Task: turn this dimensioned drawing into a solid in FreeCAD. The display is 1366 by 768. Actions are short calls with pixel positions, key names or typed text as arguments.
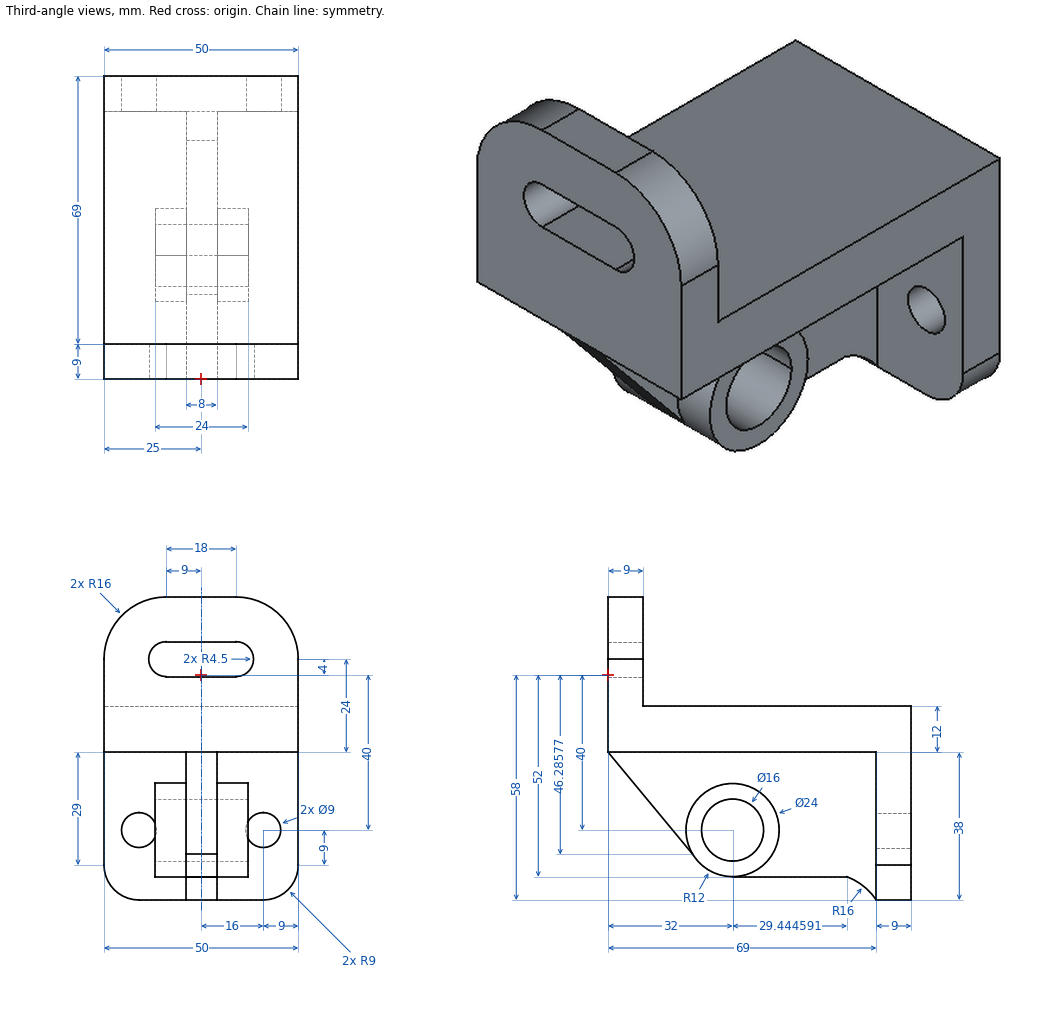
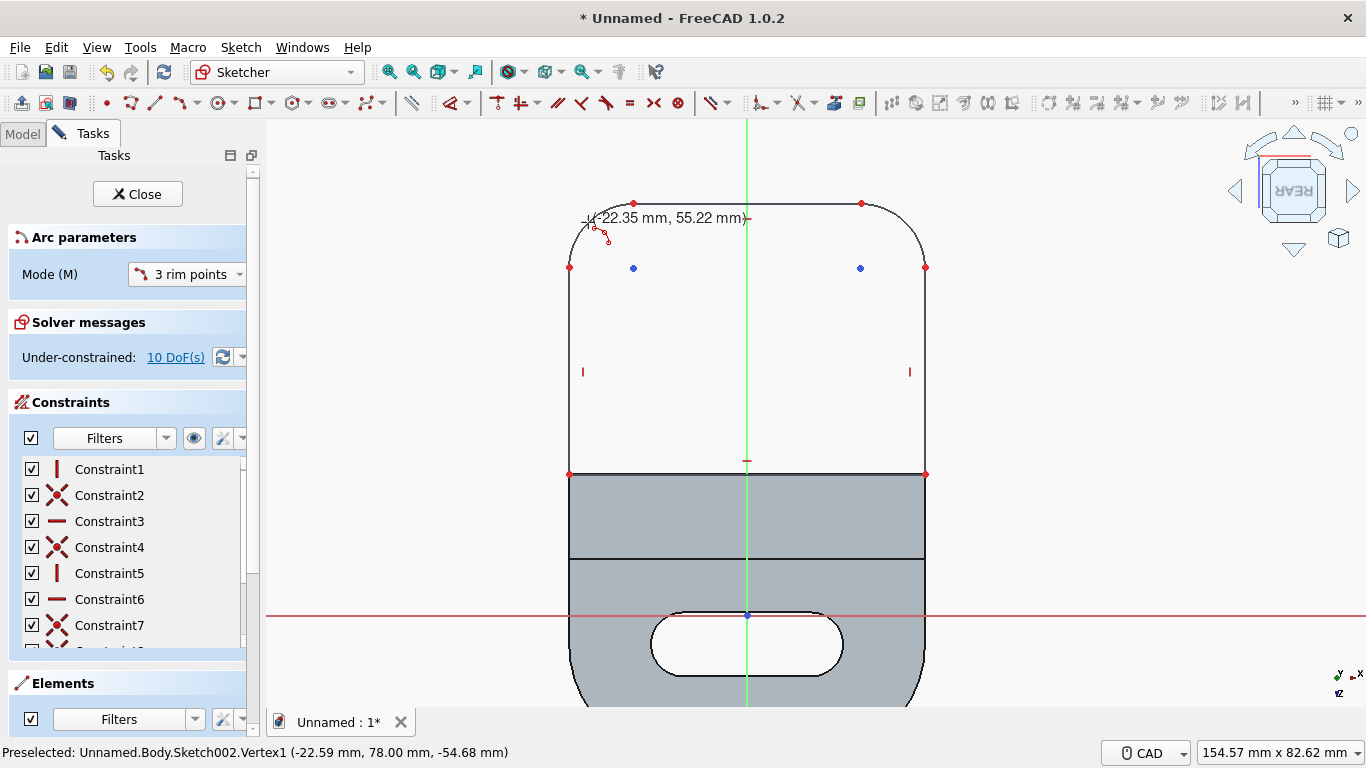
click(218, 104)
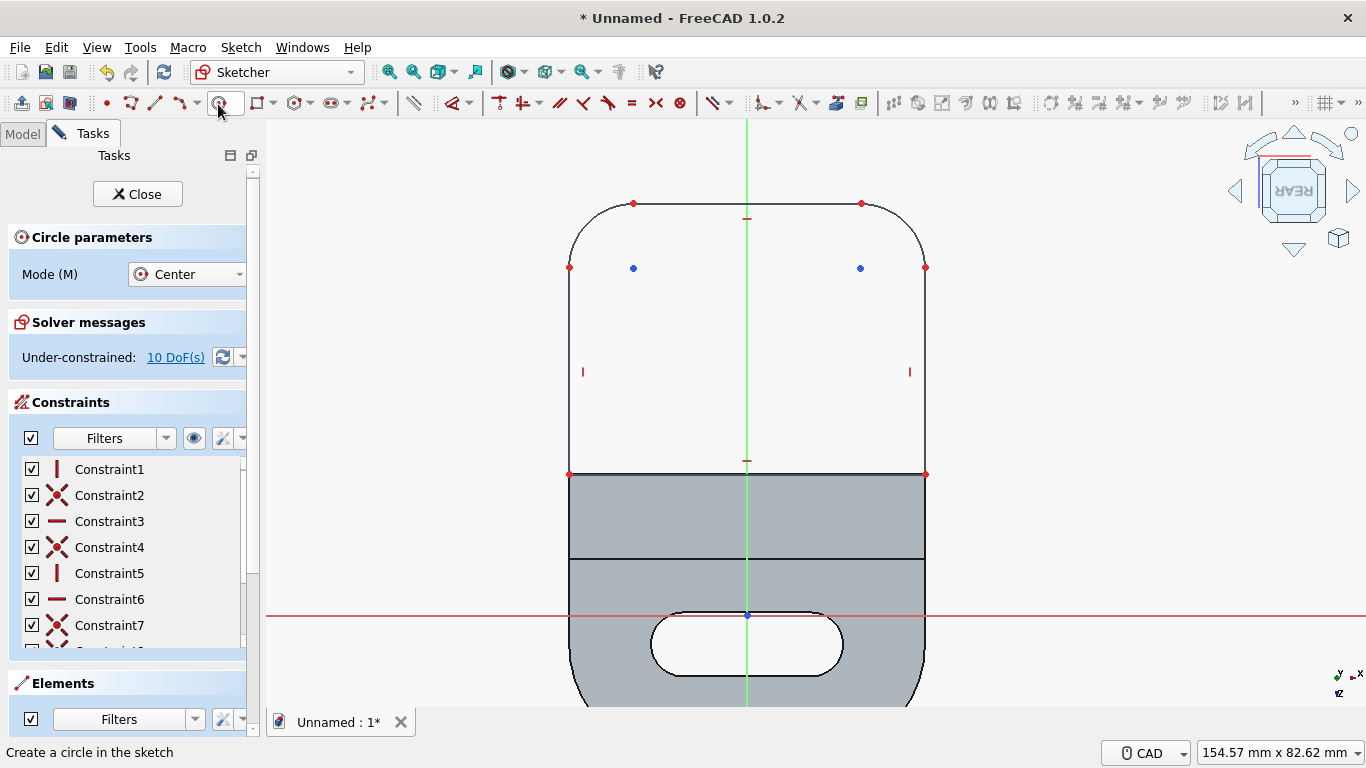
click(861, 331)
click(884, 309)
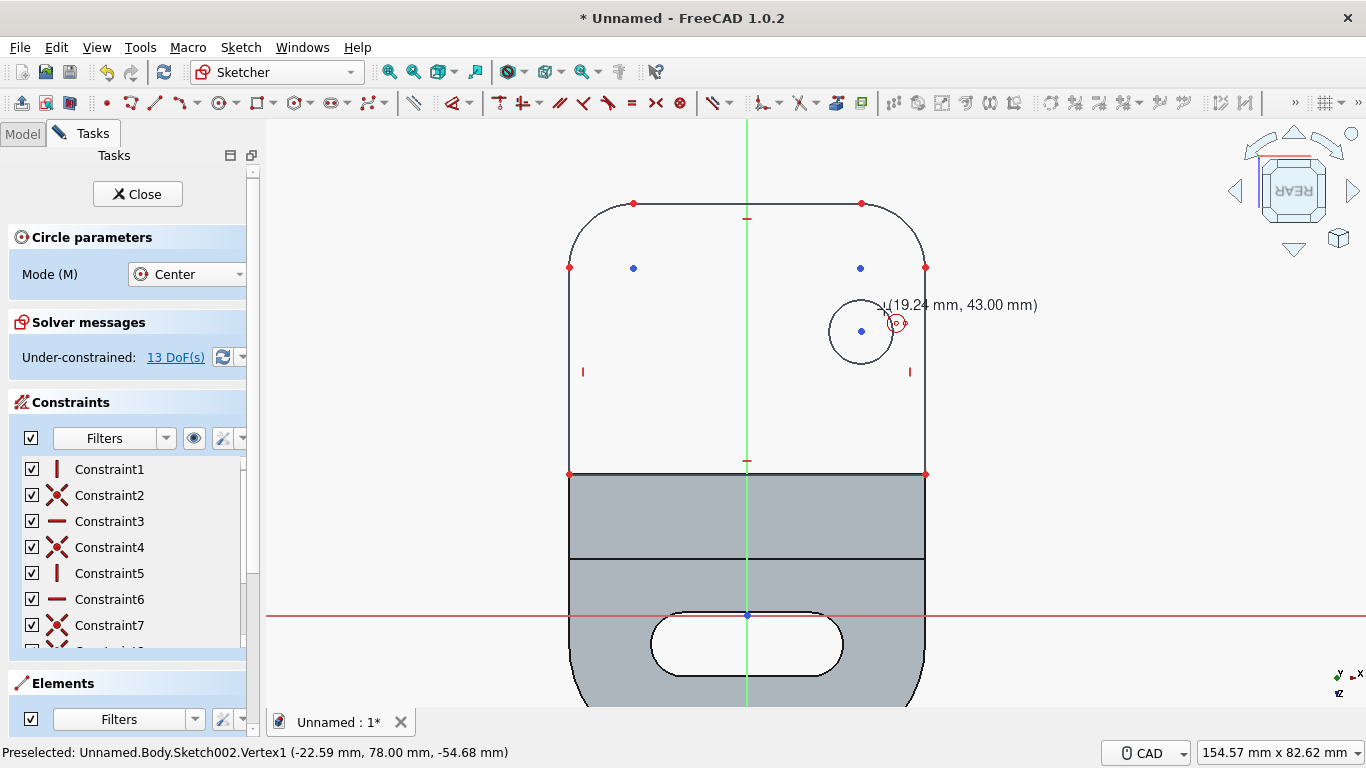
click(633, 331)
click(656, 309)
key(Escape)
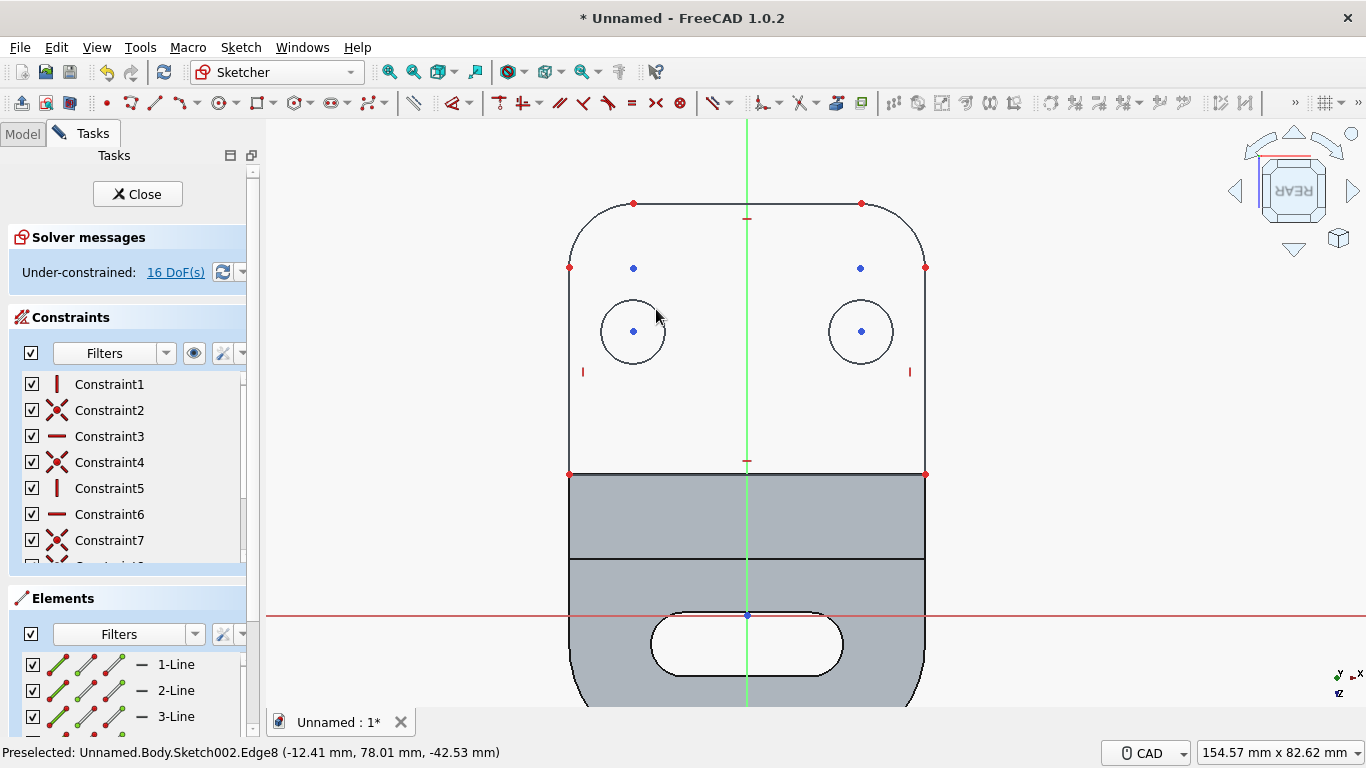
click(569, 330)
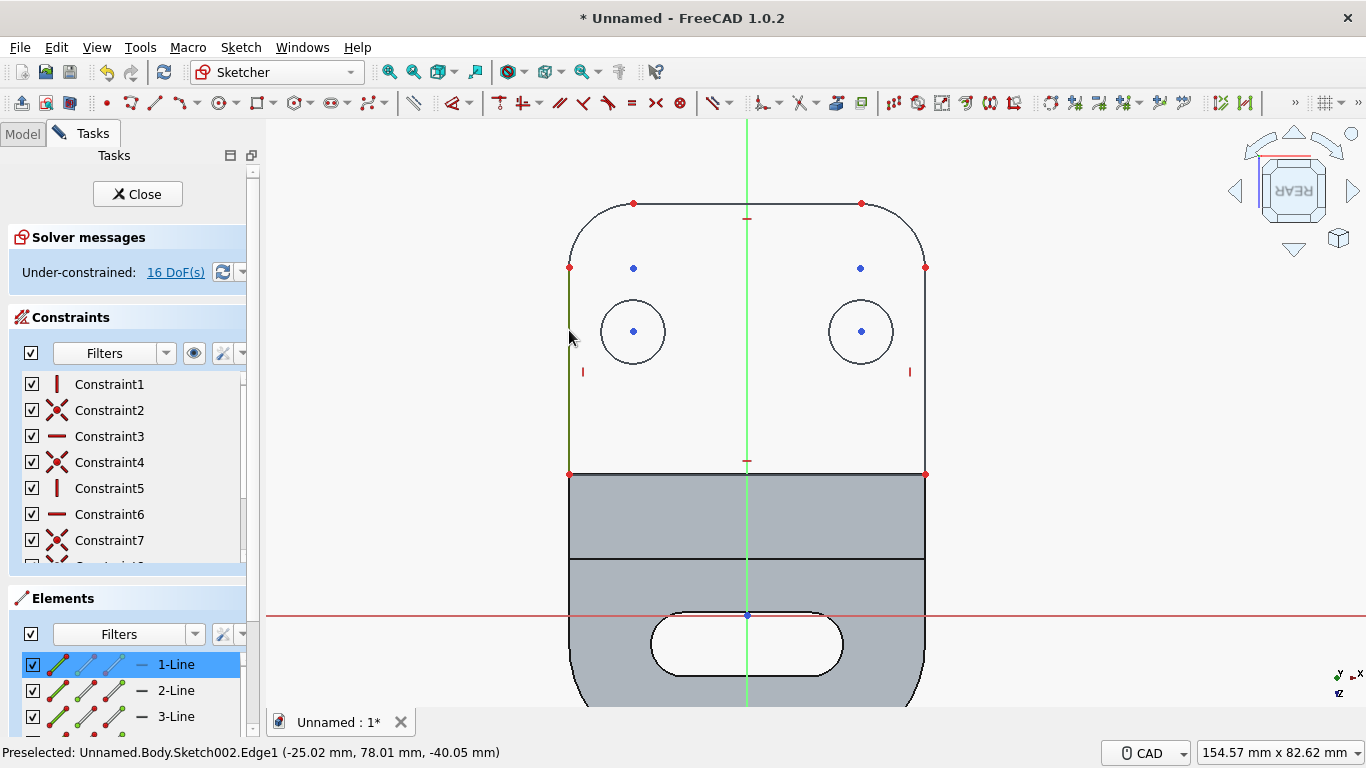
click(604, 211)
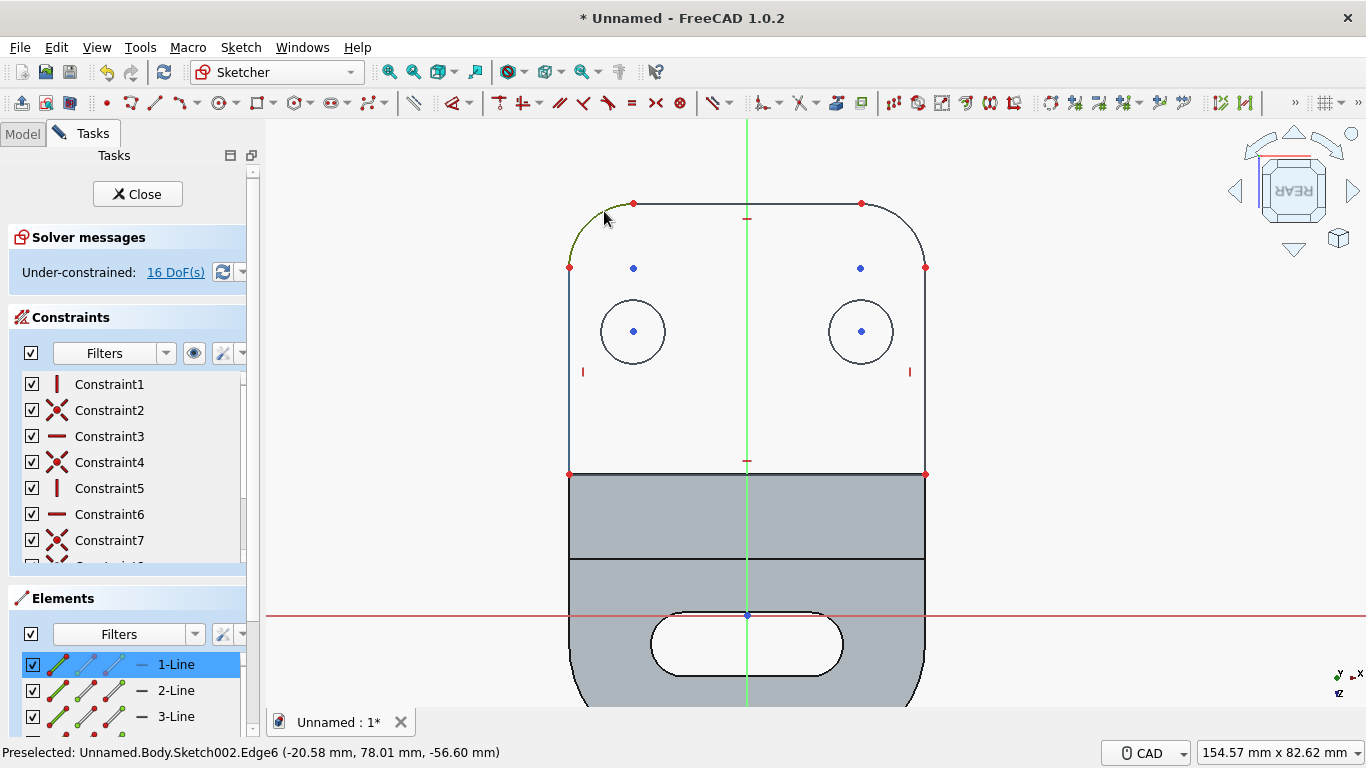
click(608, 104)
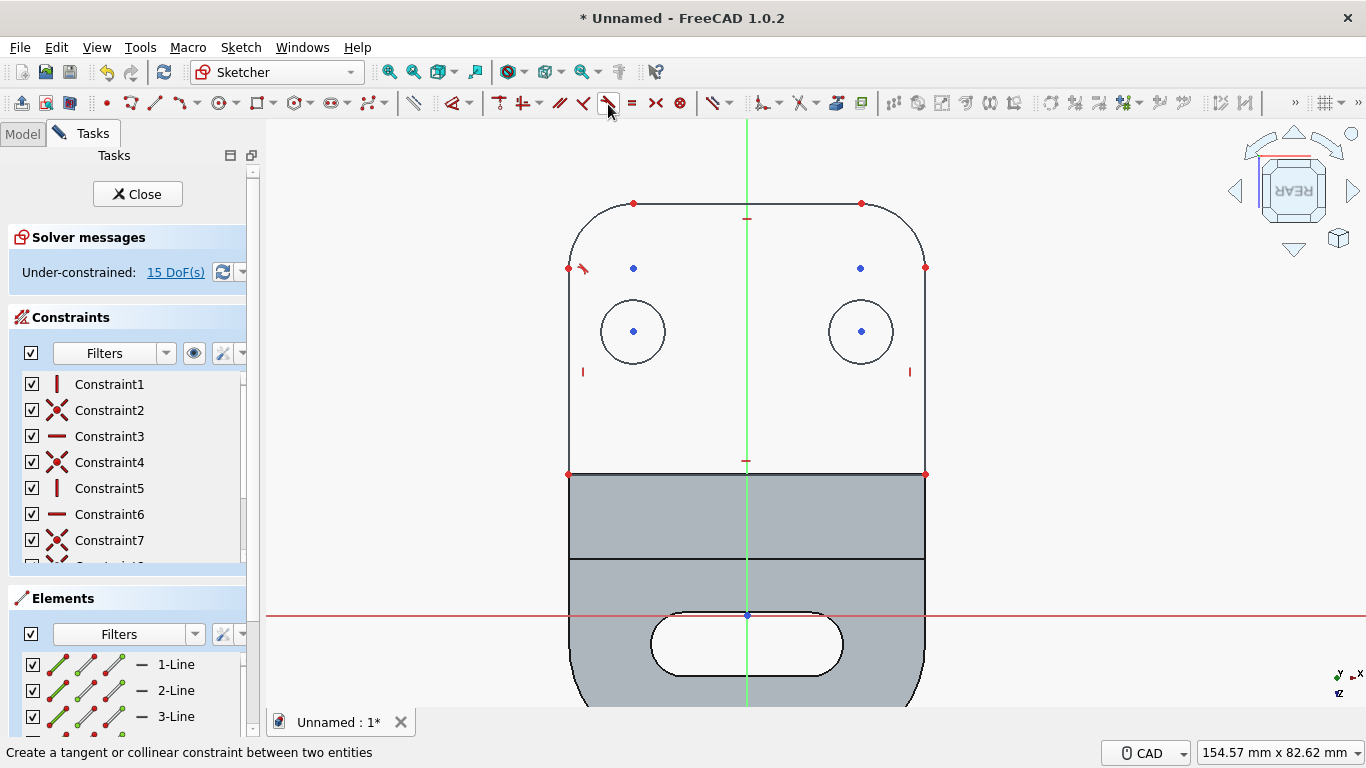
click(925, 413)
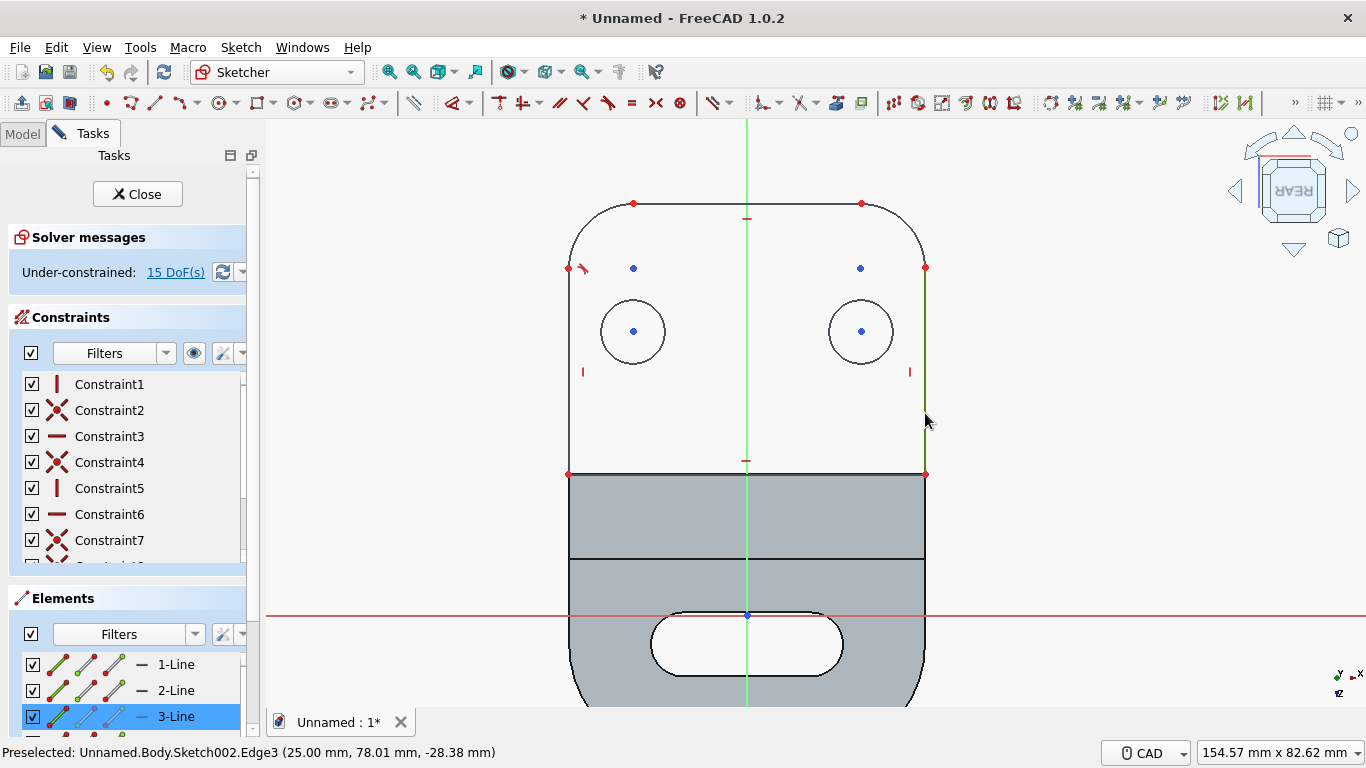
click(918, 239)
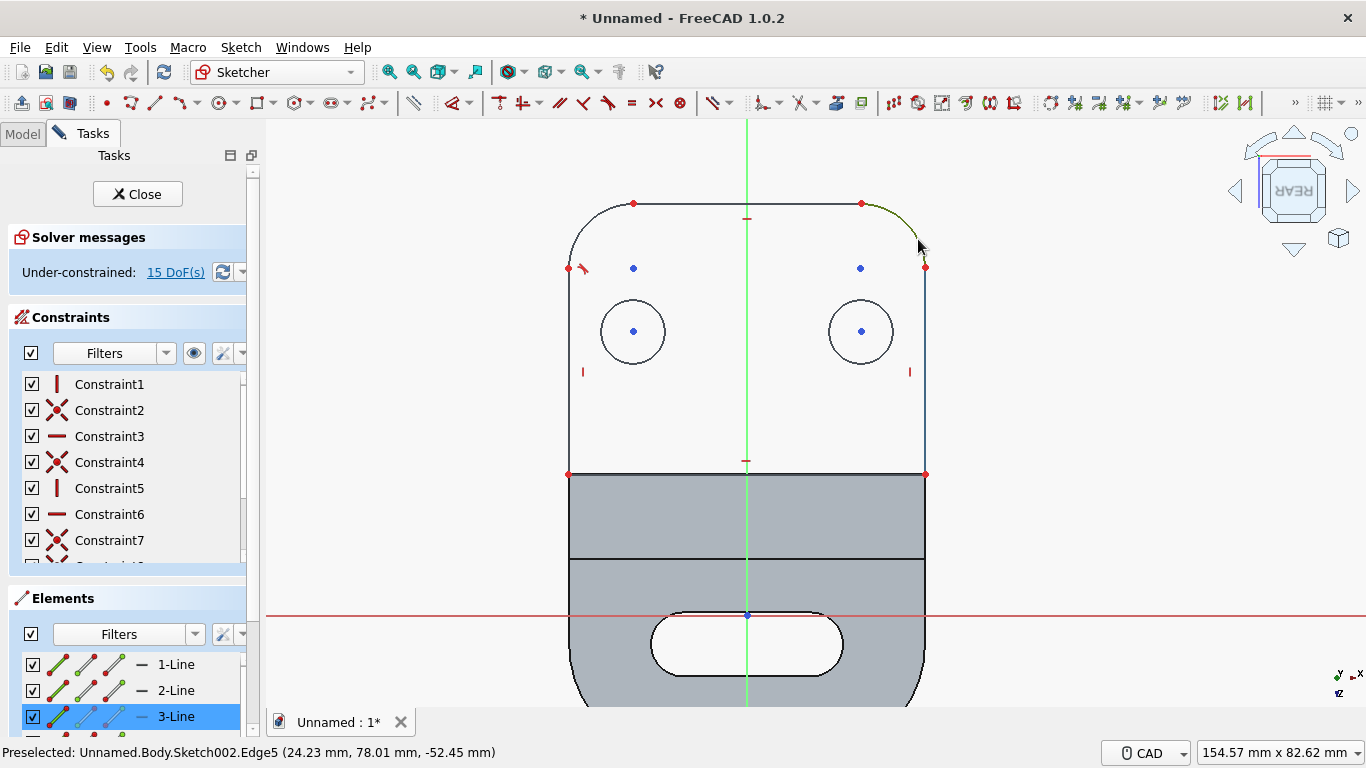
click(608, 104)